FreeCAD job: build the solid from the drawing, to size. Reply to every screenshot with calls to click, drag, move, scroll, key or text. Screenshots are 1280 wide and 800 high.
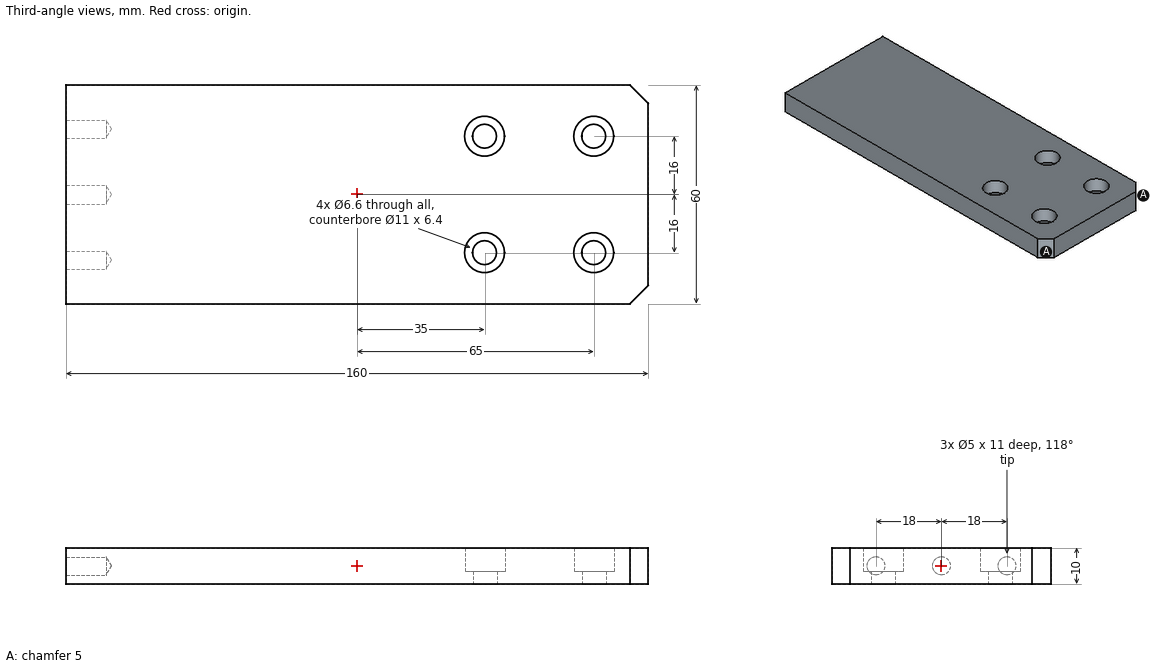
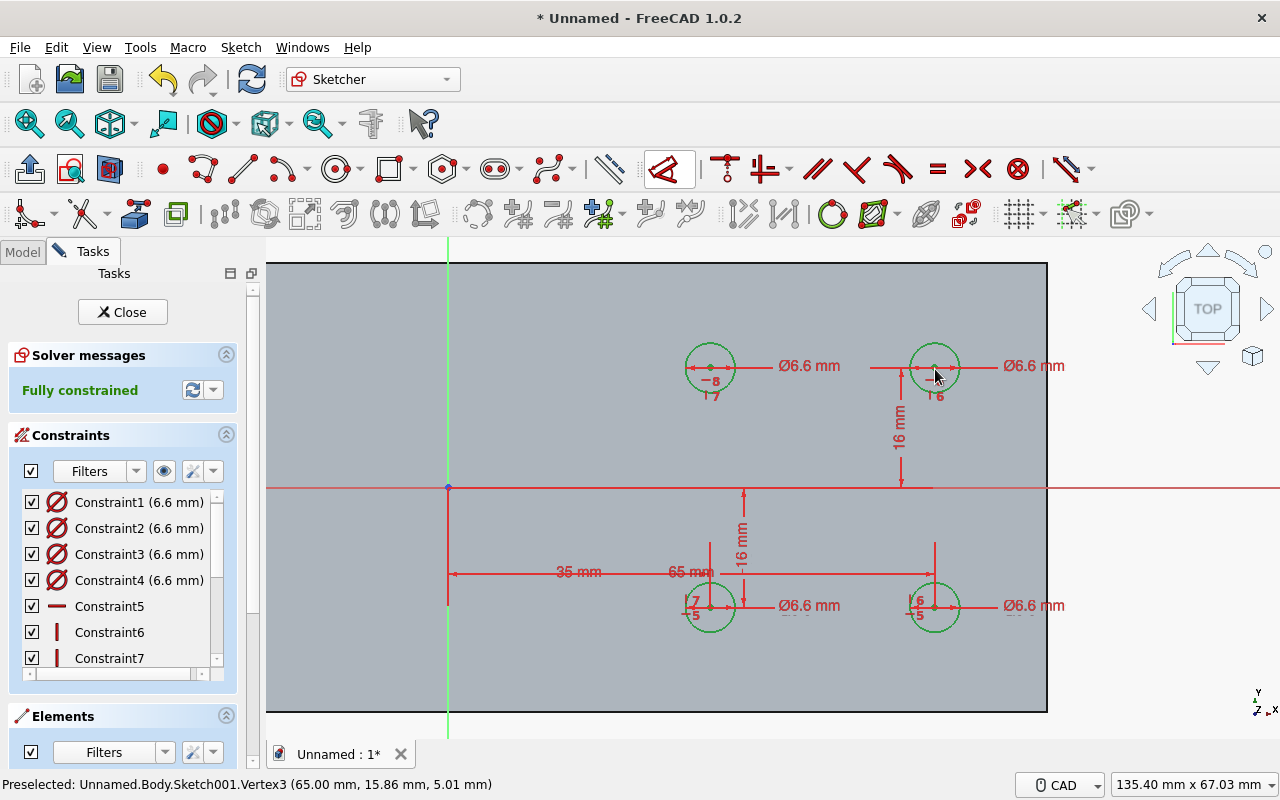
click(123, 312)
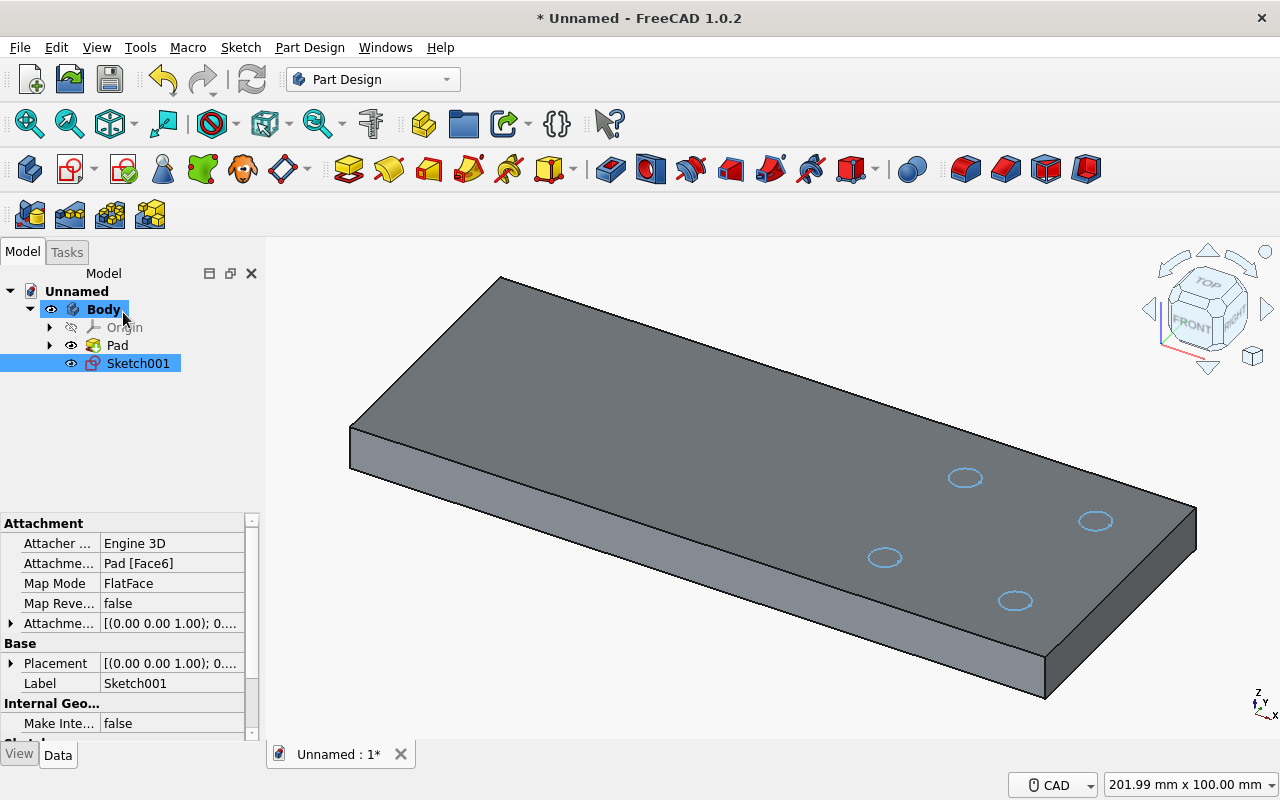
click(652, 170)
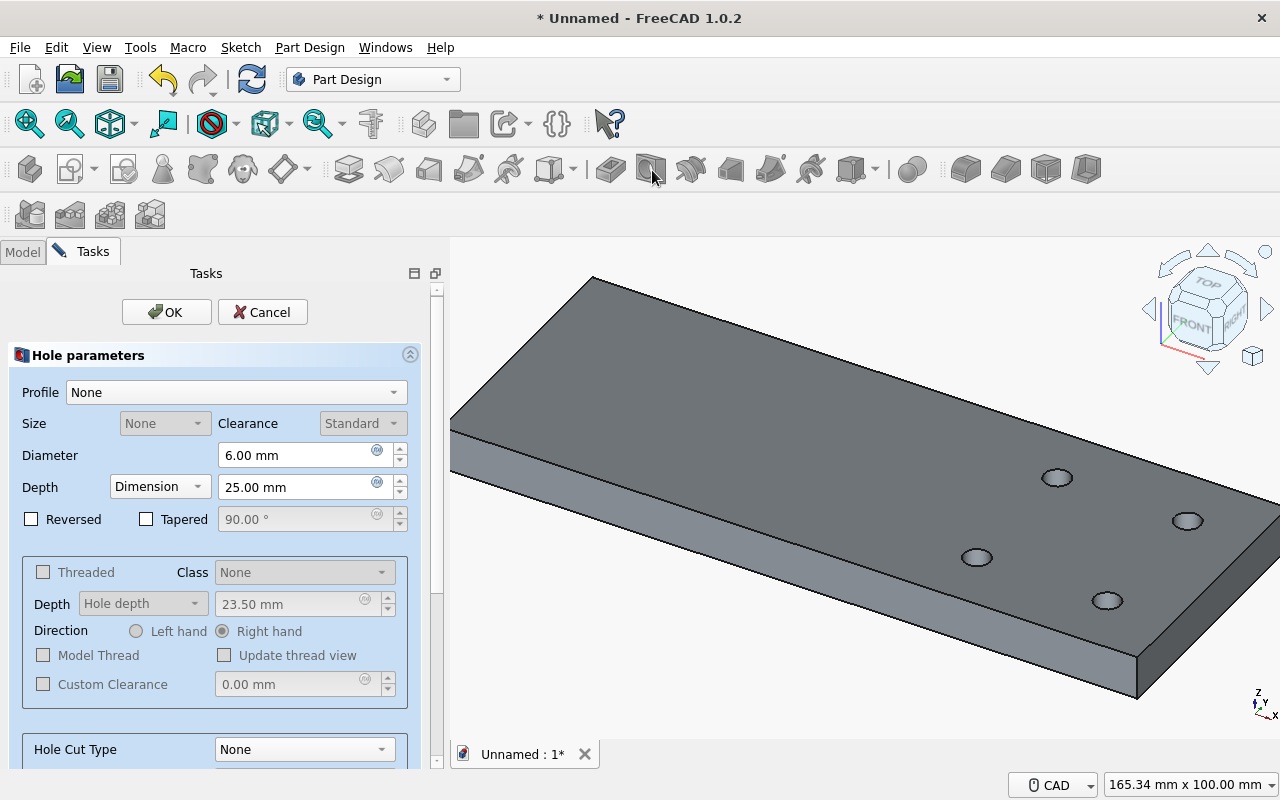
triple_click(305, 455)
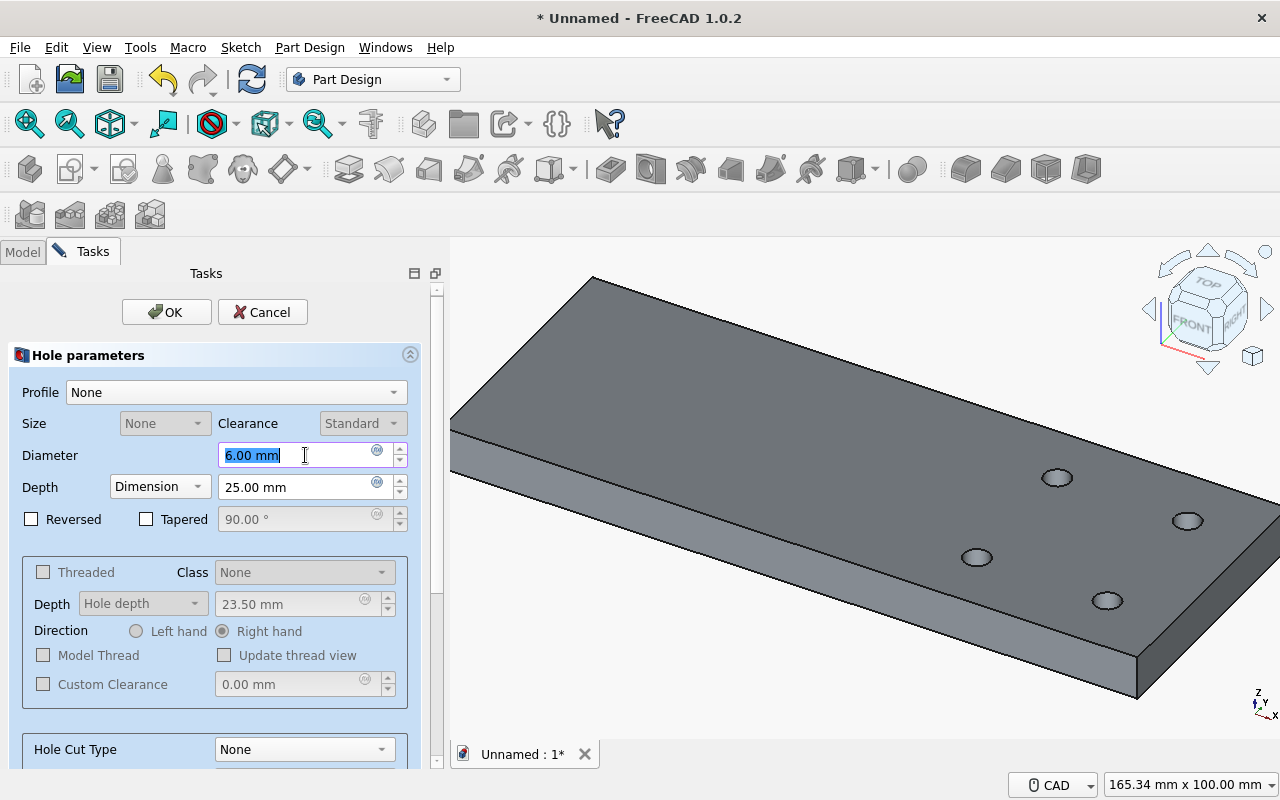
text(6.6)
key(Tab)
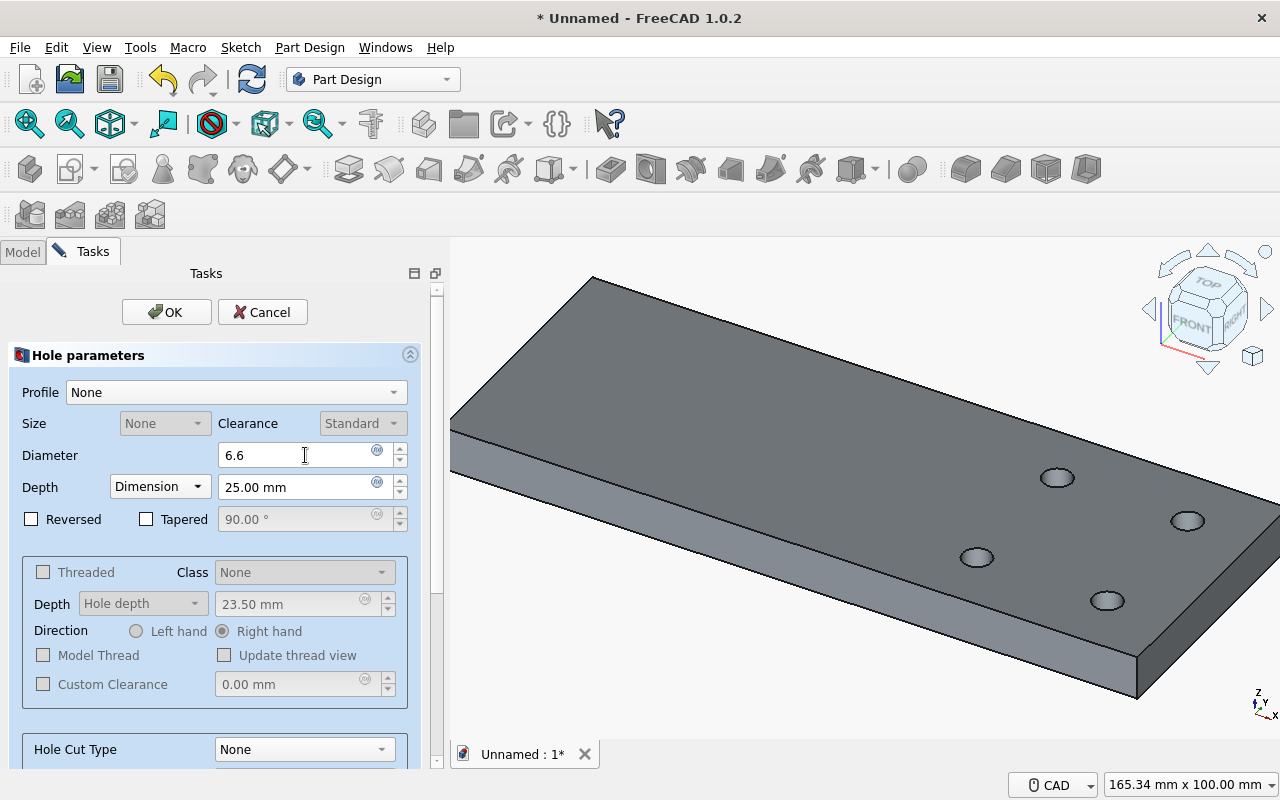
click(161, 486)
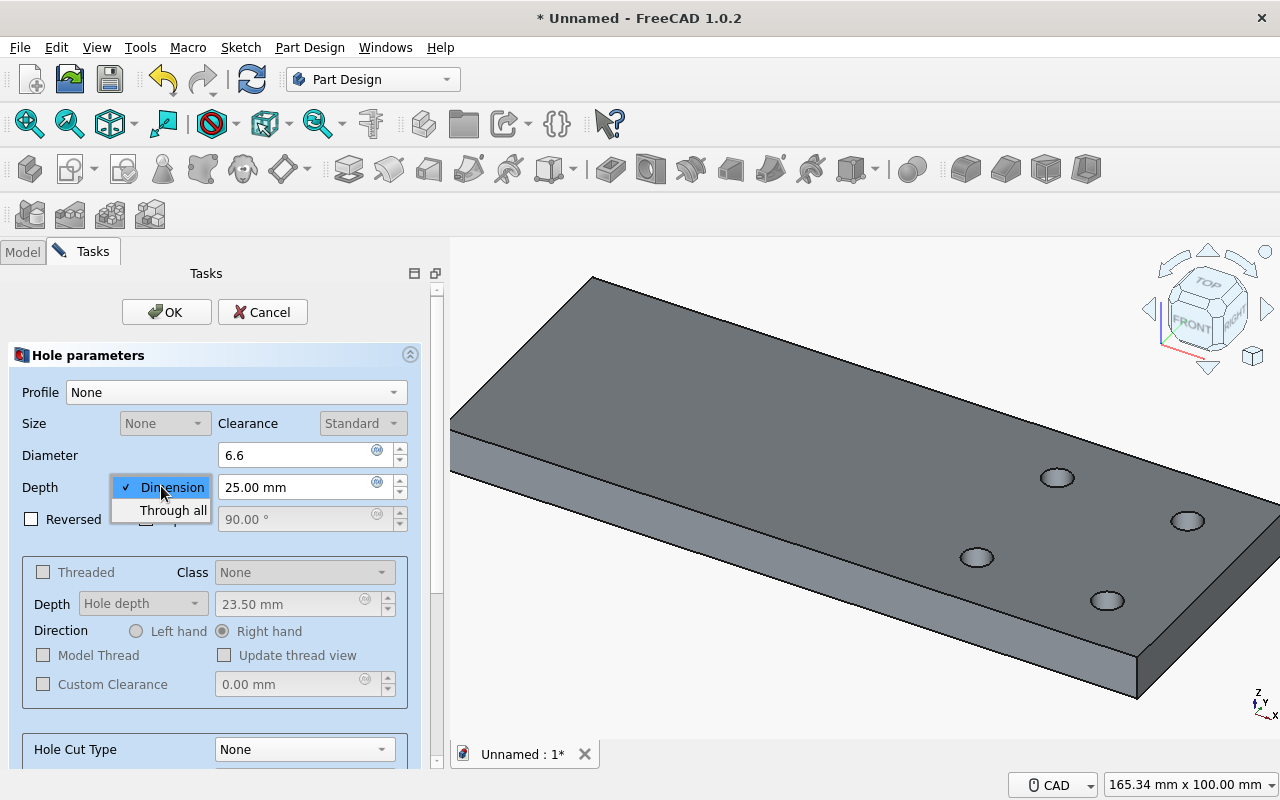
click(160, 510)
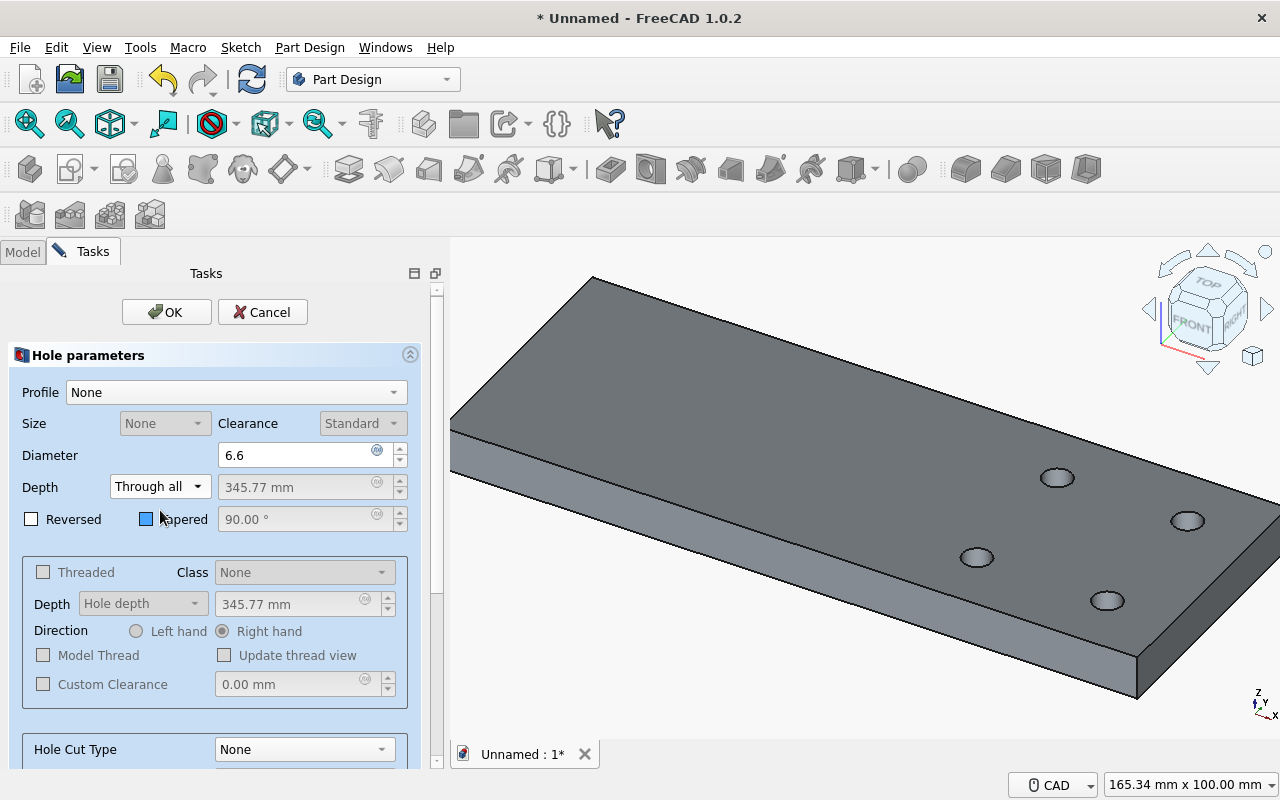
click(306, 750)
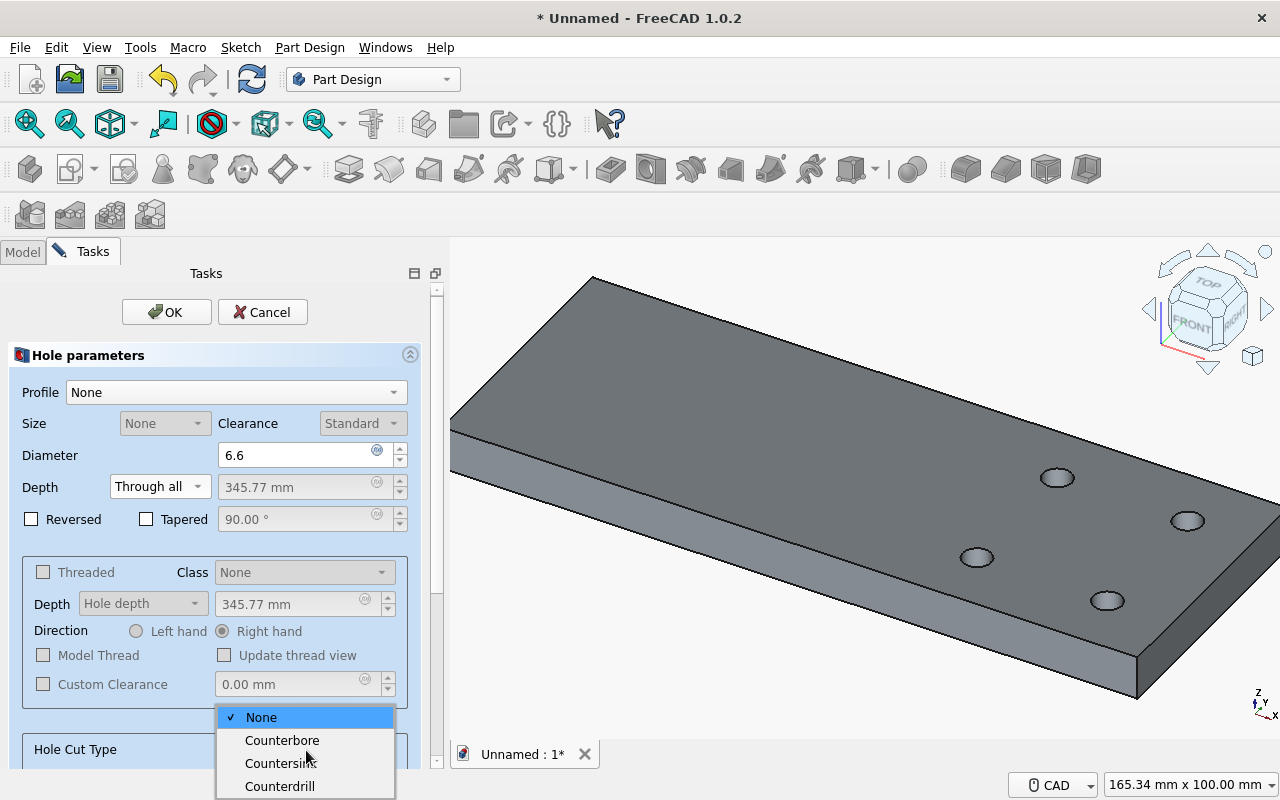
click(304, 740)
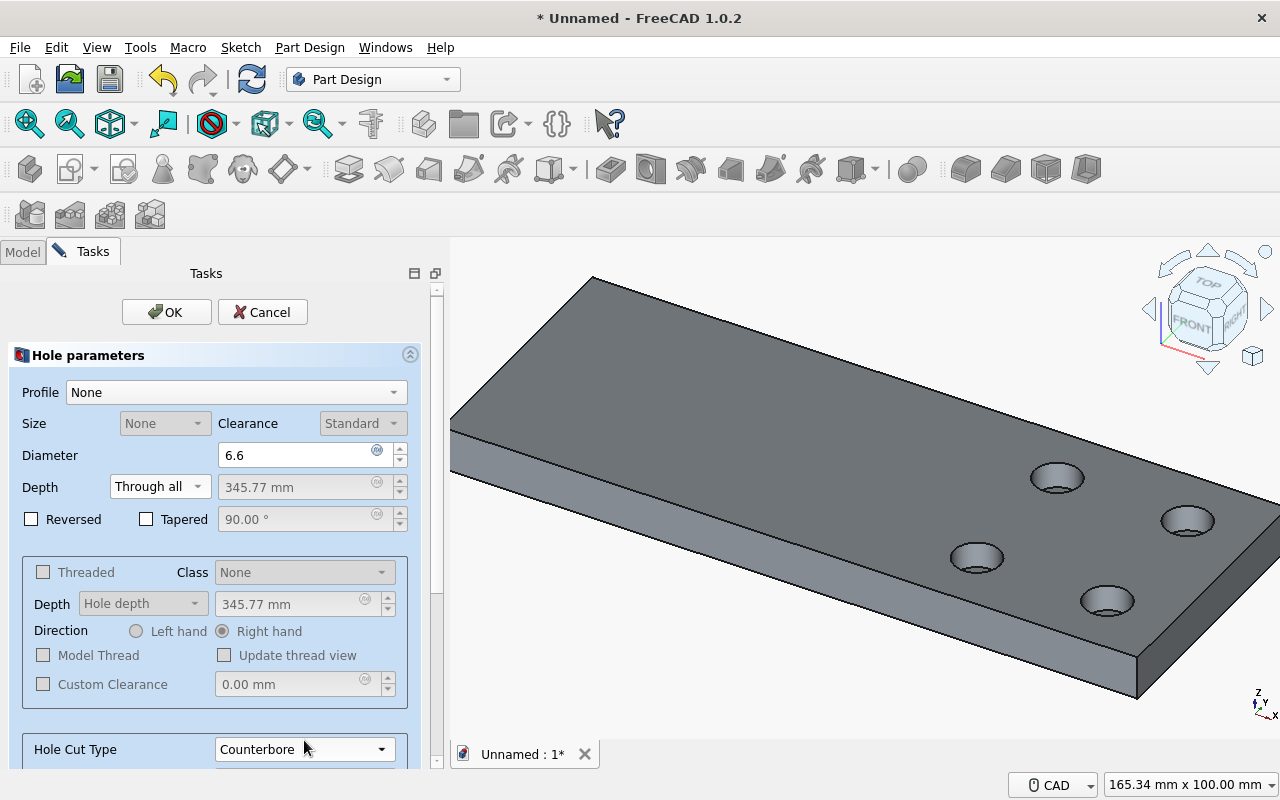
scroll(437, 526, down, 2)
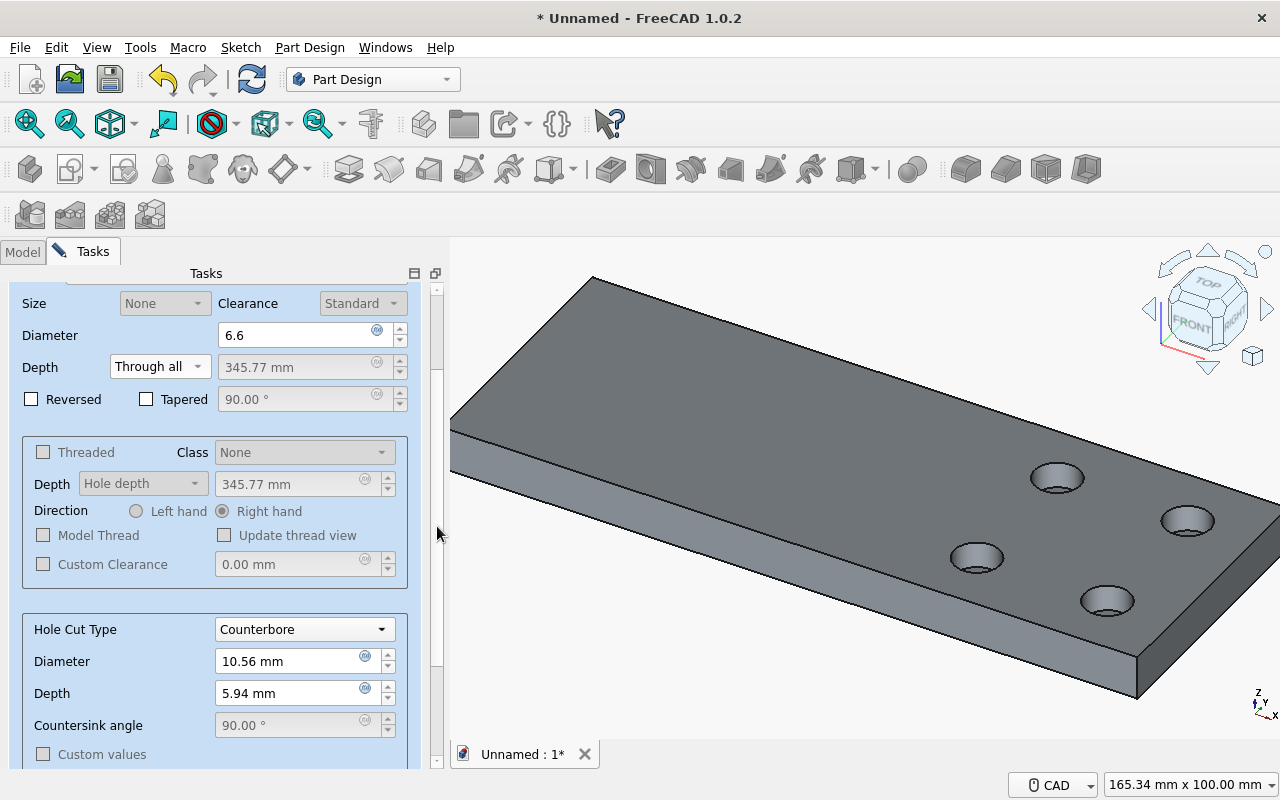
triple_click(298, 661)